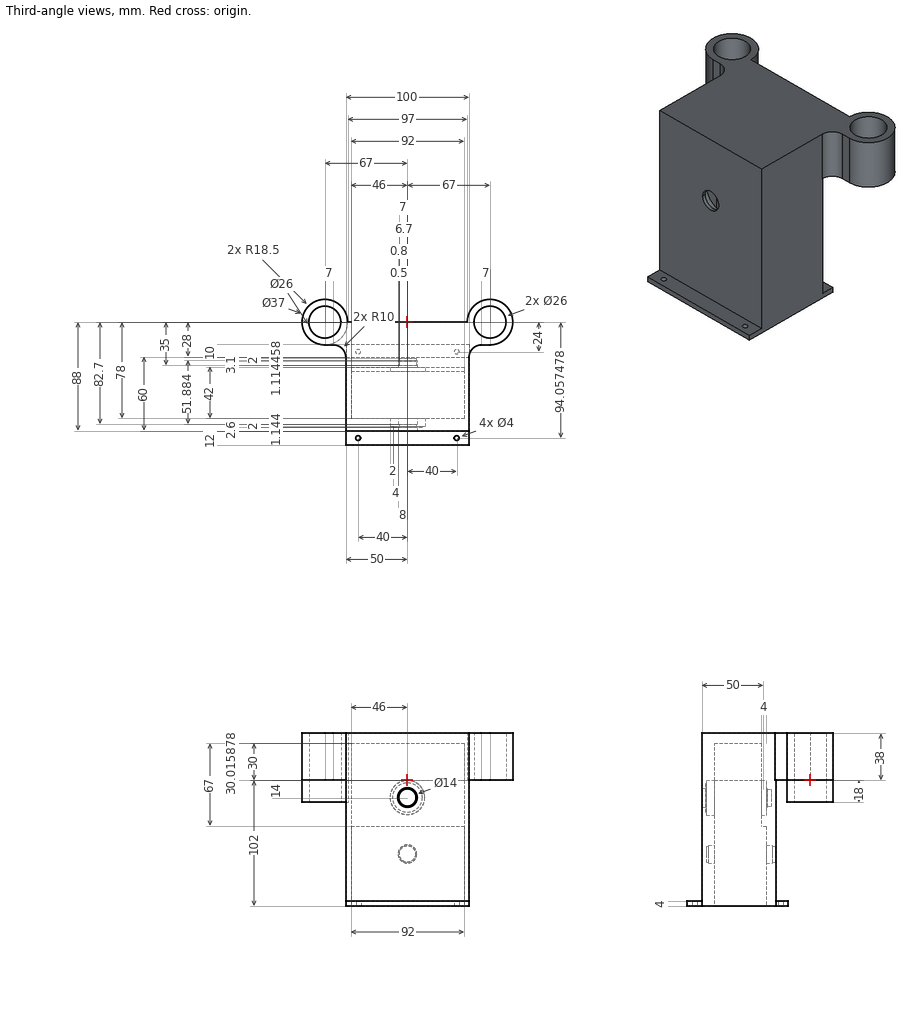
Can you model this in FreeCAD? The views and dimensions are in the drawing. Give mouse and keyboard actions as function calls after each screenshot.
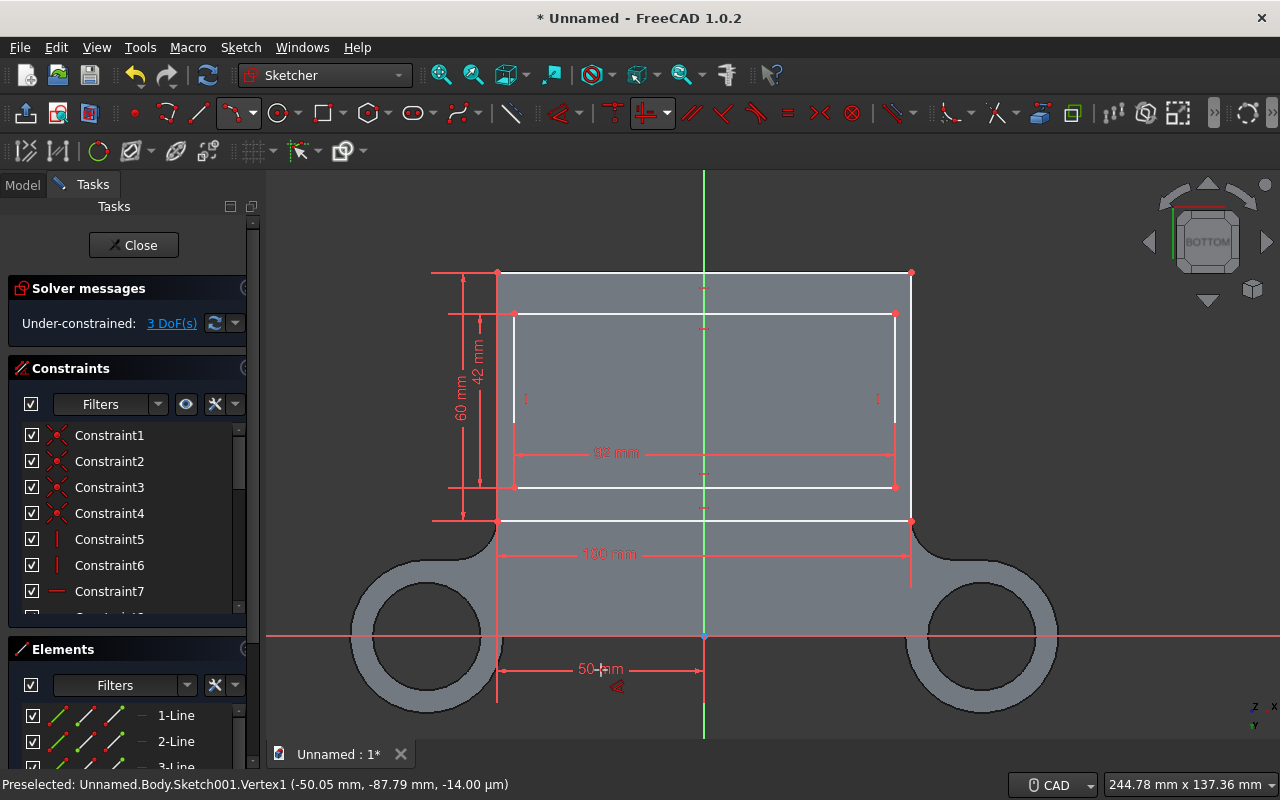
click(497, 273)
click(463, 455)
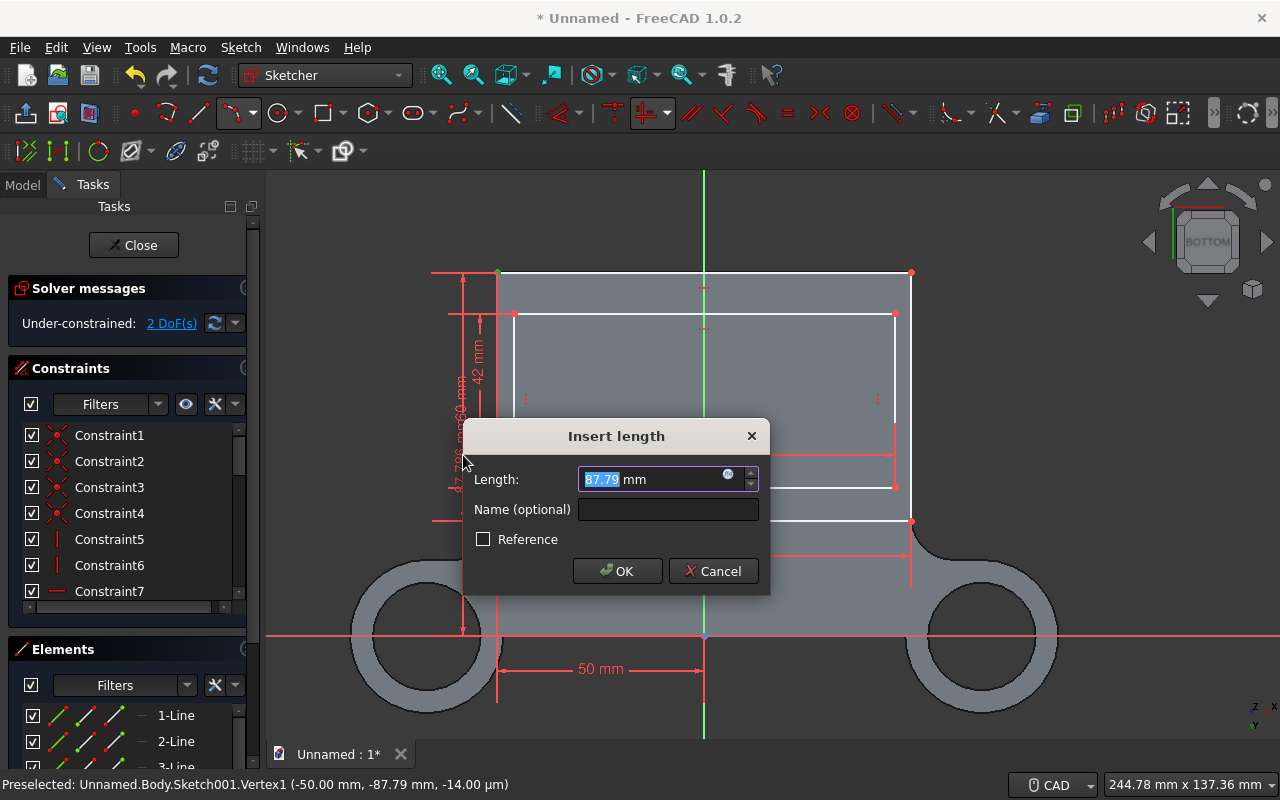
text(88)
key(Return)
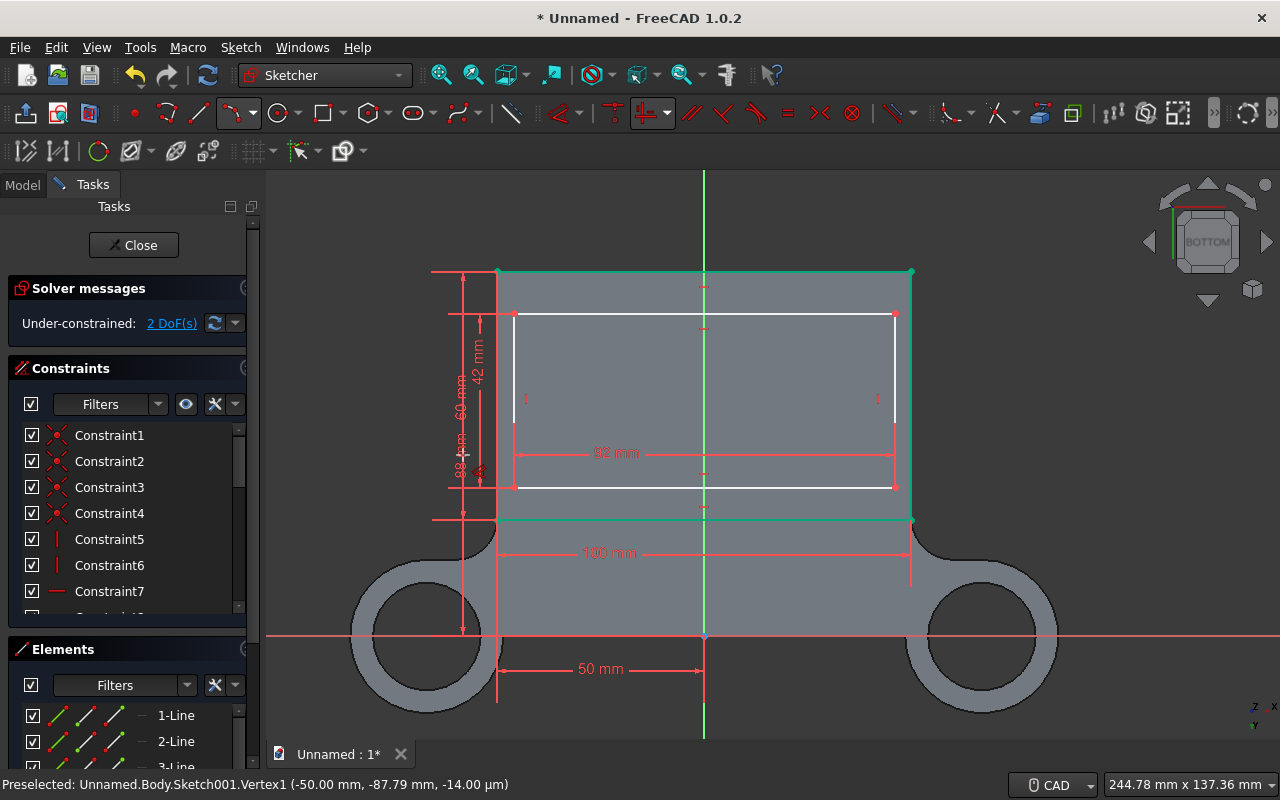
click(514, 314)
click(676, 670)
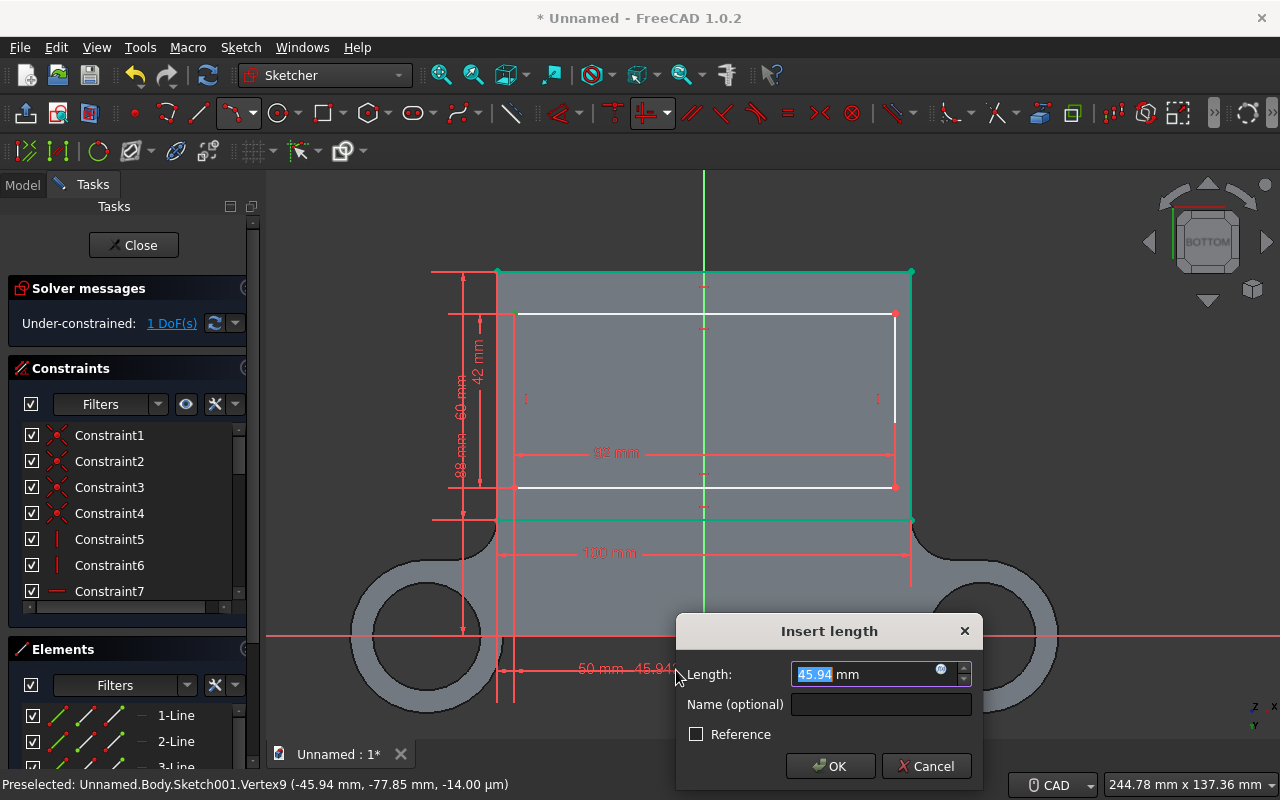
text(46)
key(Return)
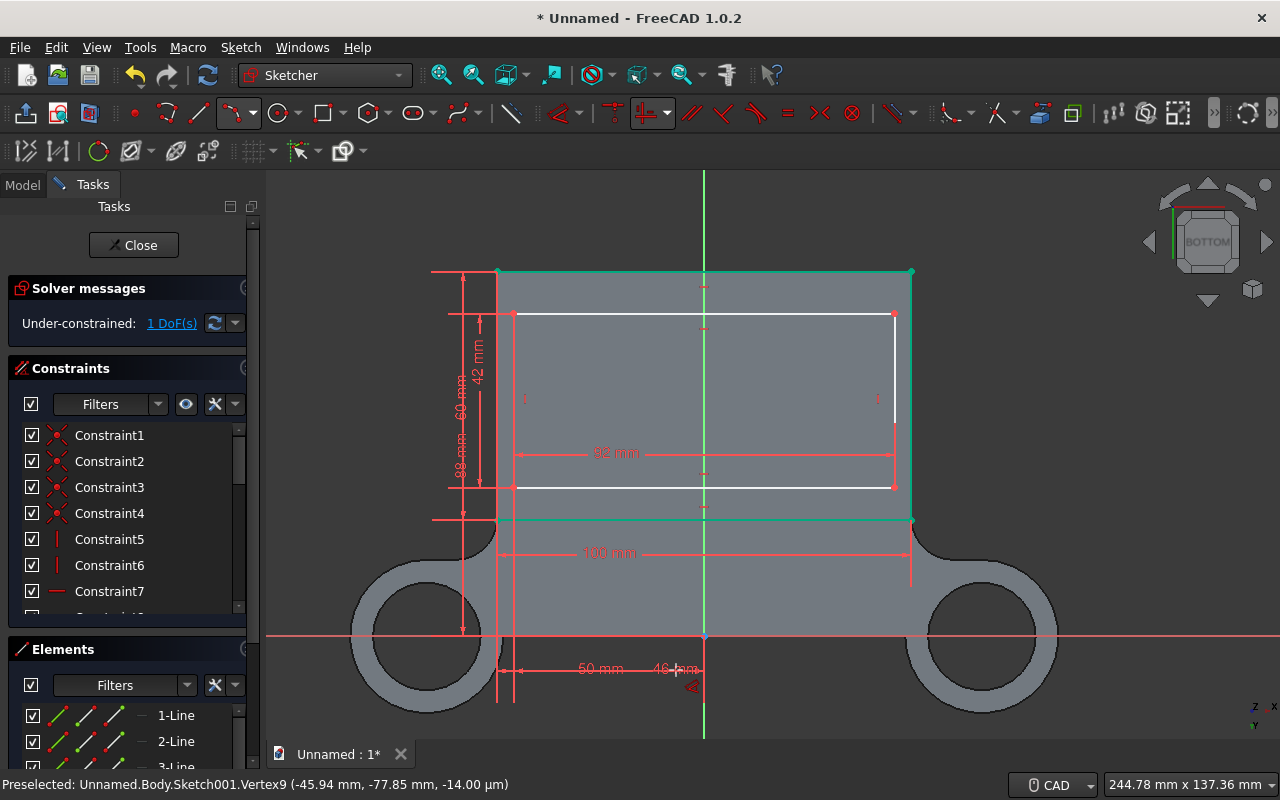
click(514, 314)
click(480, 475)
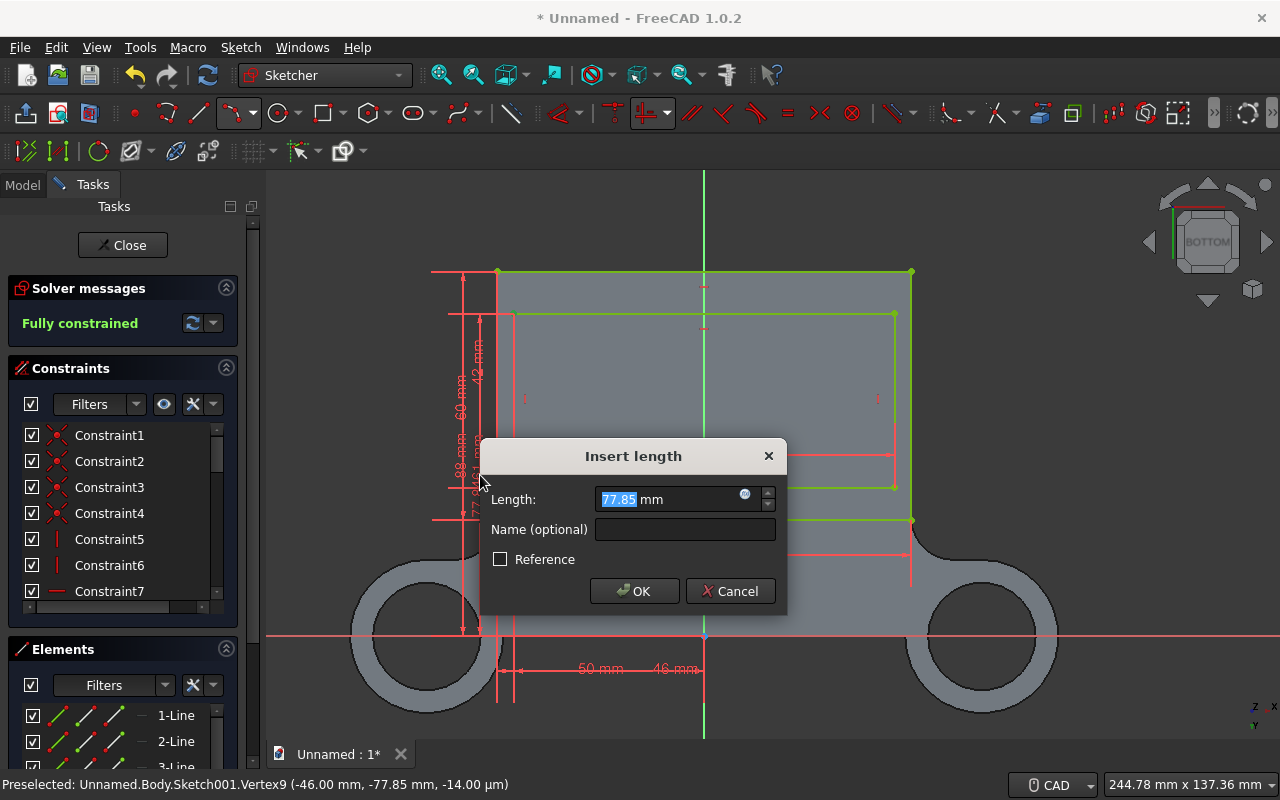
text(78)
key(Return)
key(Escape)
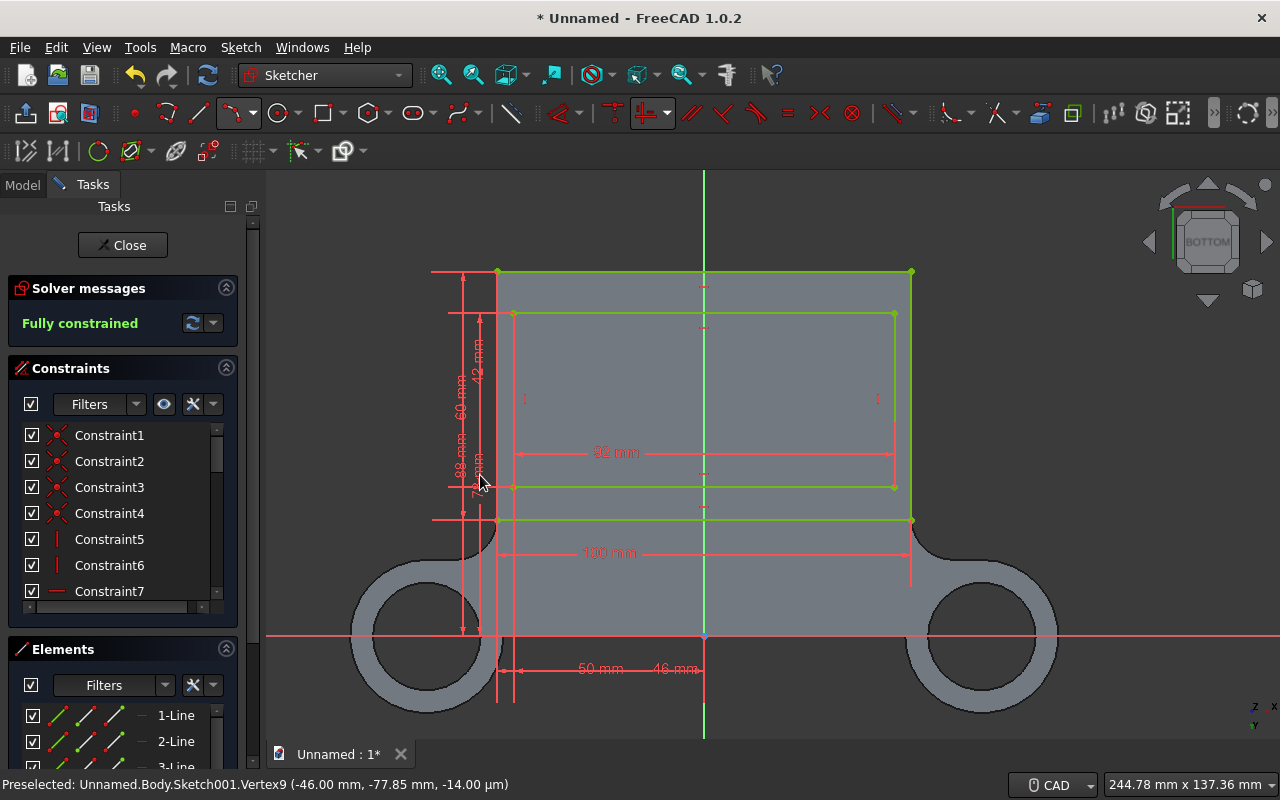
click(123, 245)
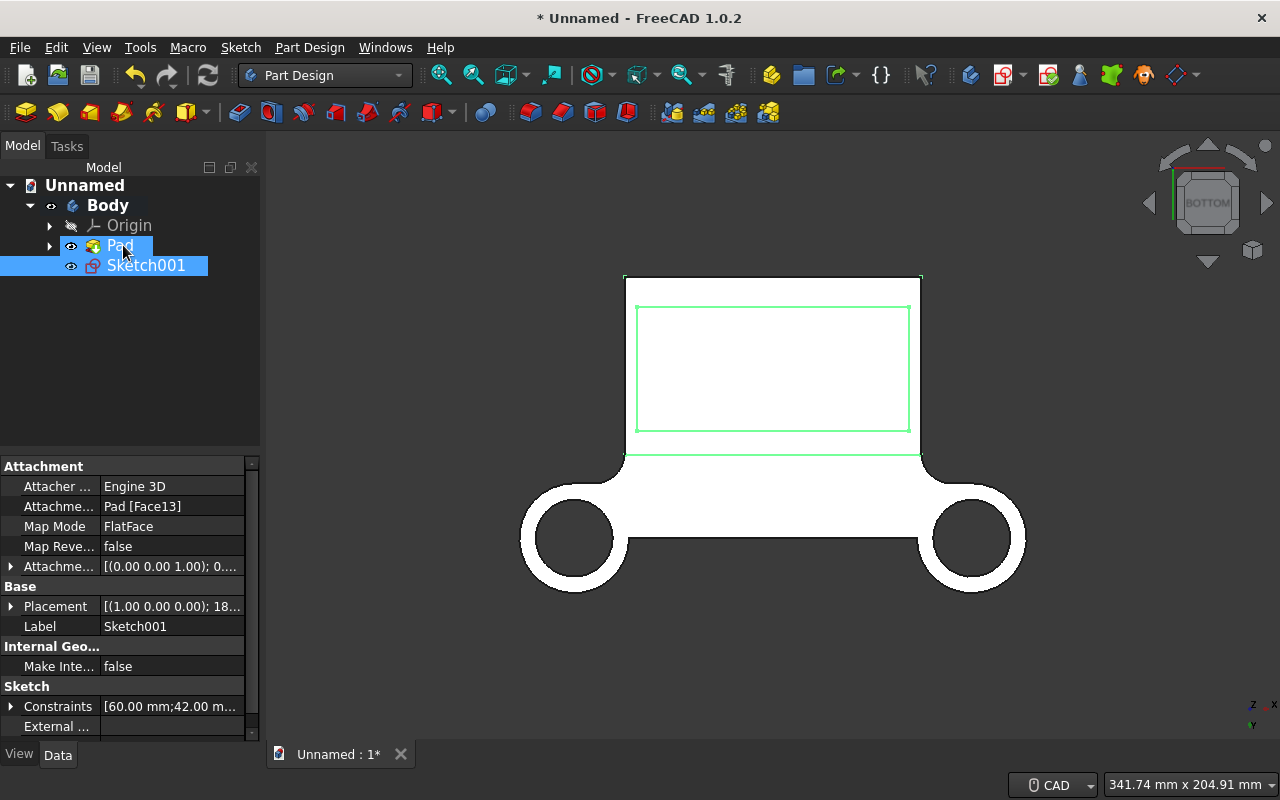
click(26, 112)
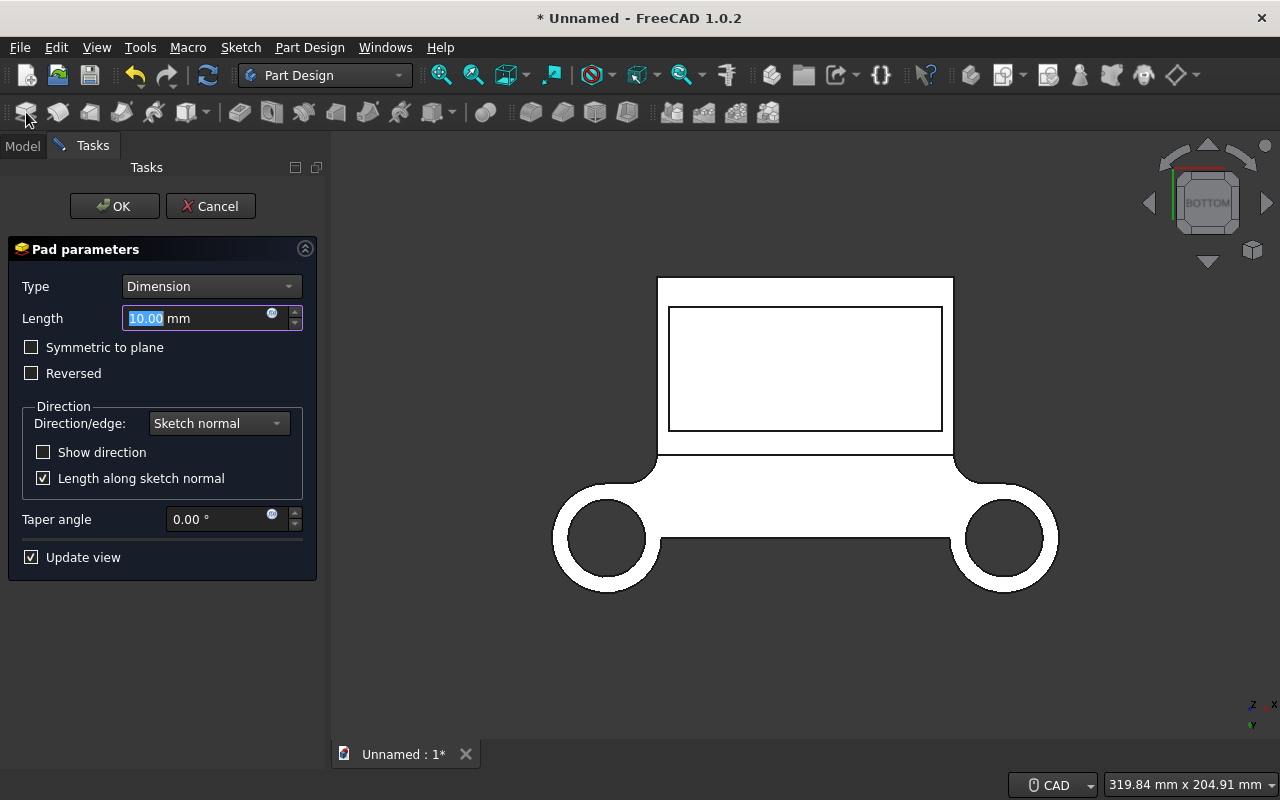
text(102)
key(Tab)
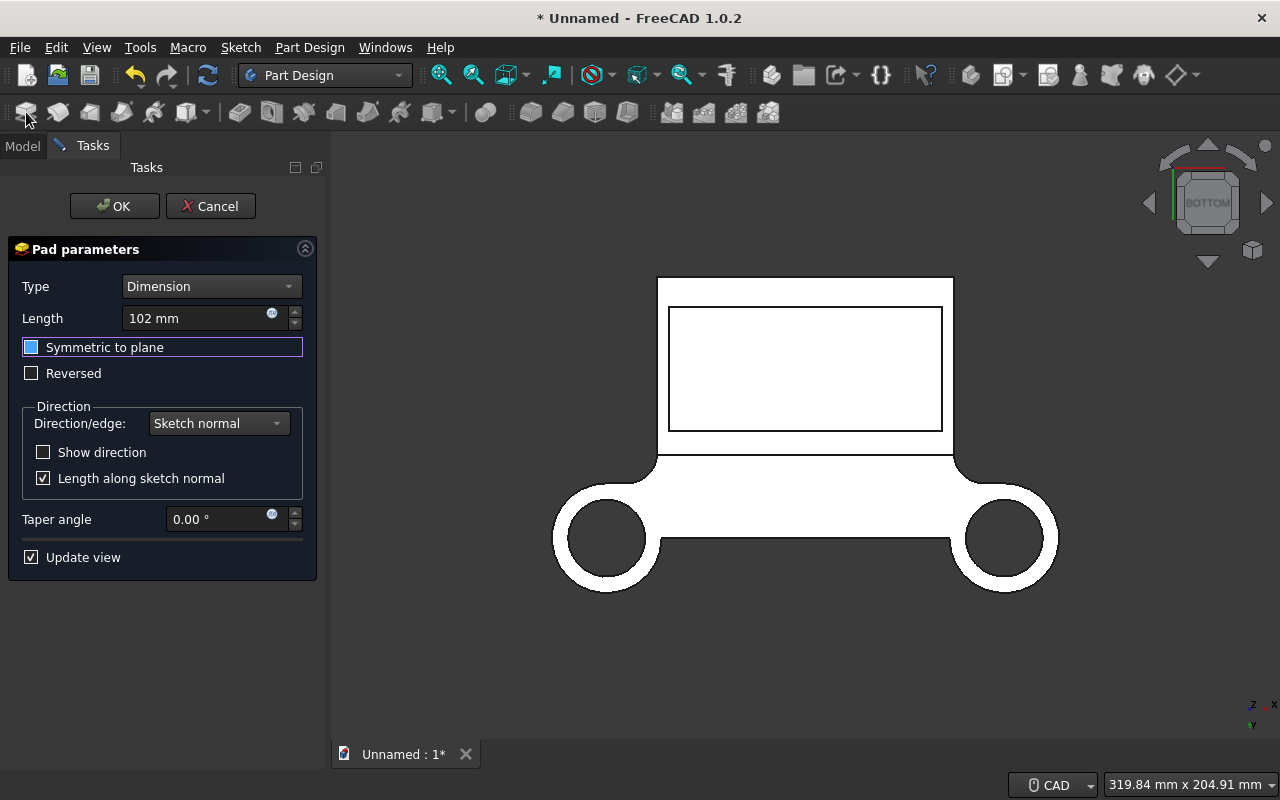
click(115, 206)